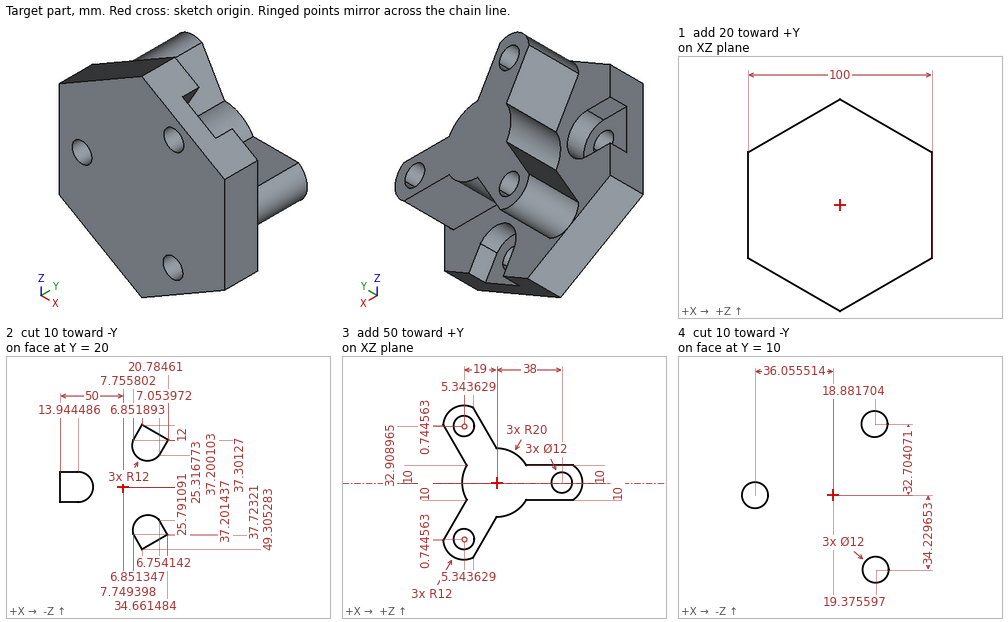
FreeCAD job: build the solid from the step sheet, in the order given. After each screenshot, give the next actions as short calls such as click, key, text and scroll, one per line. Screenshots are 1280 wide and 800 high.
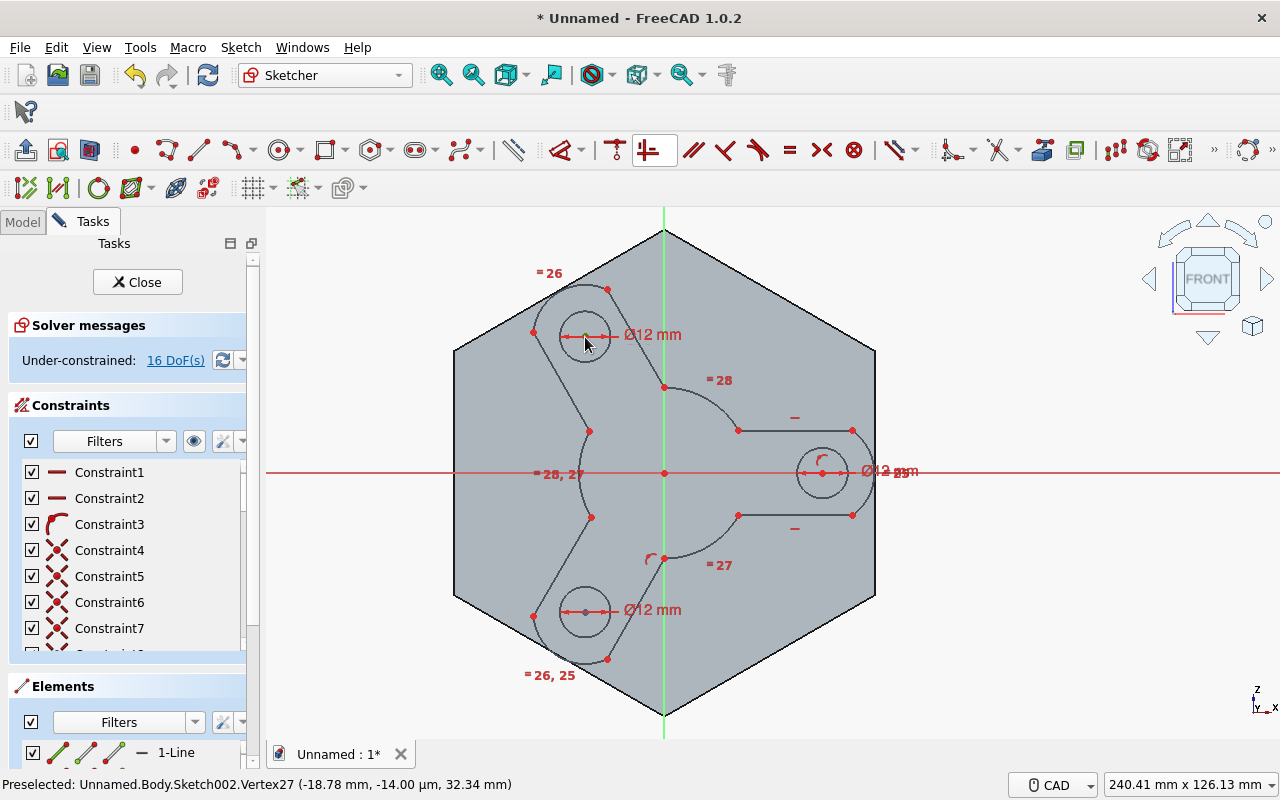
click(353, 473)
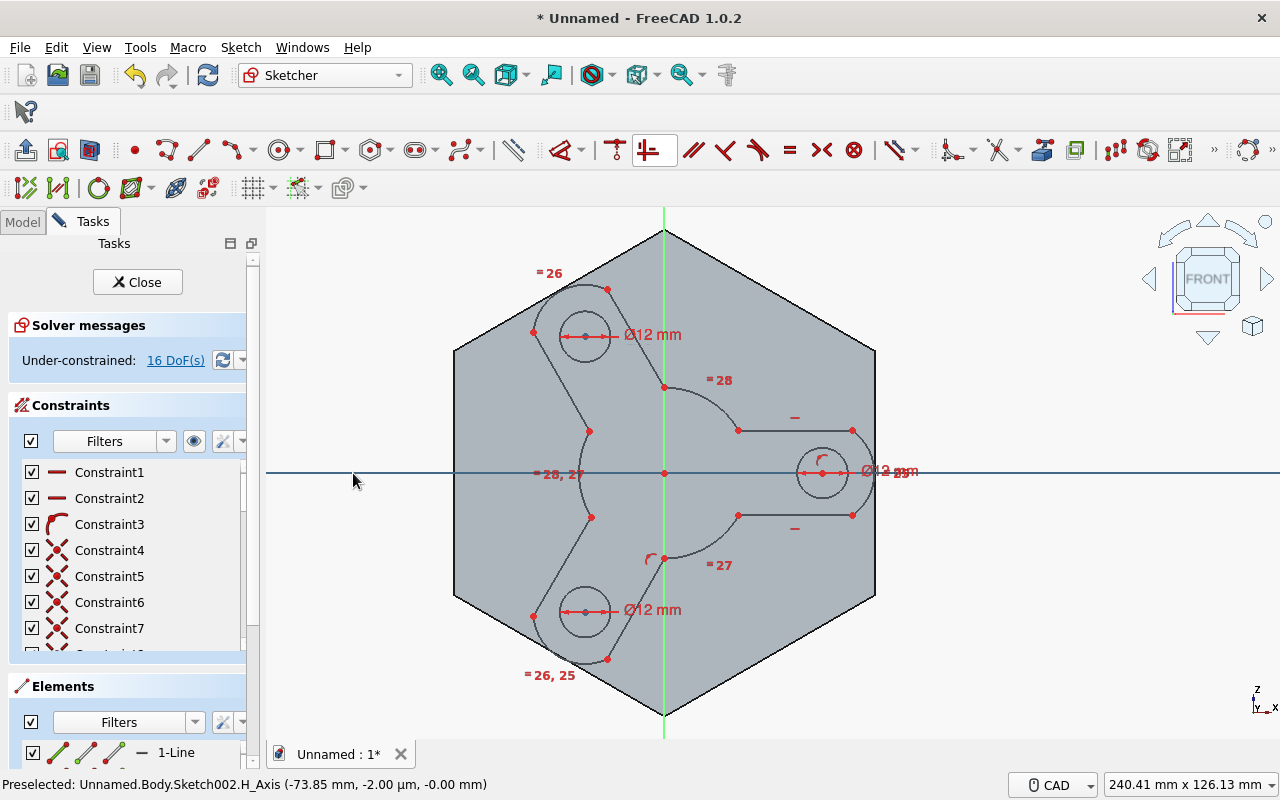
click(822, 150)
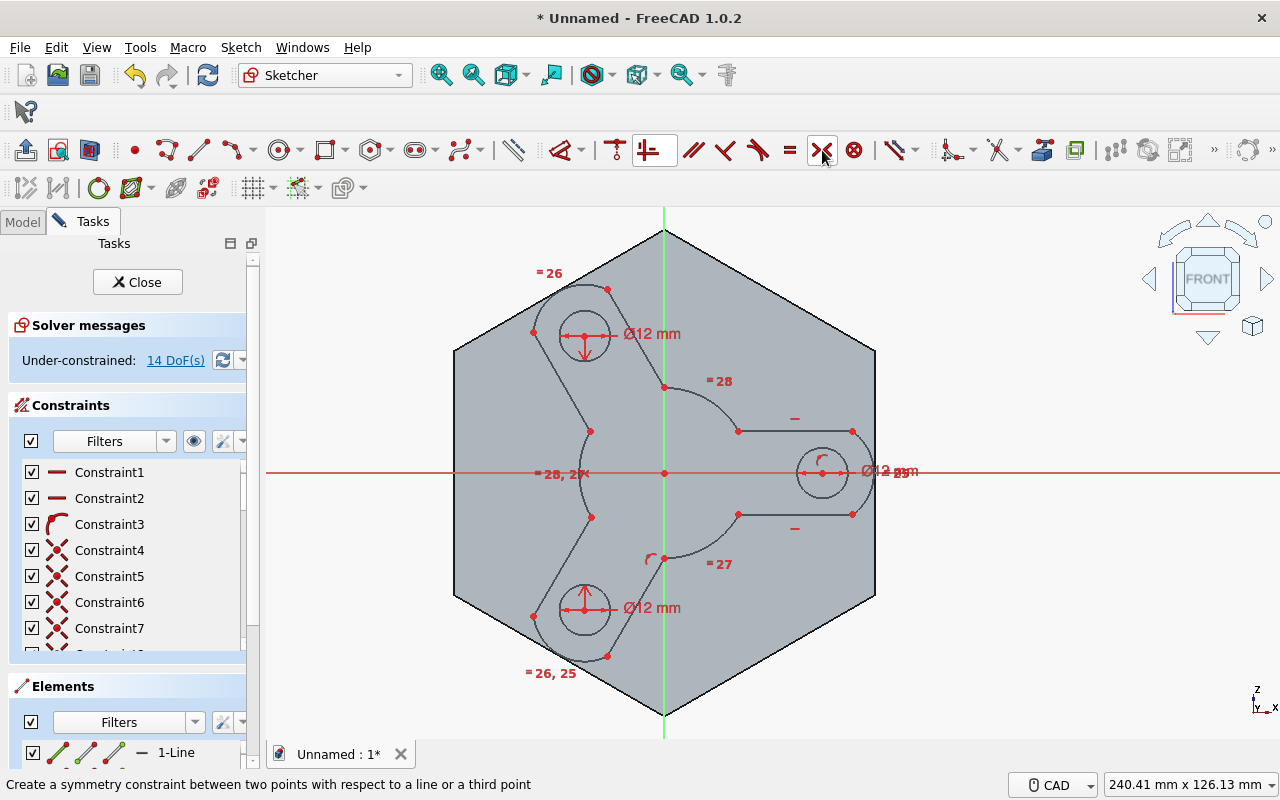
click(560, 150)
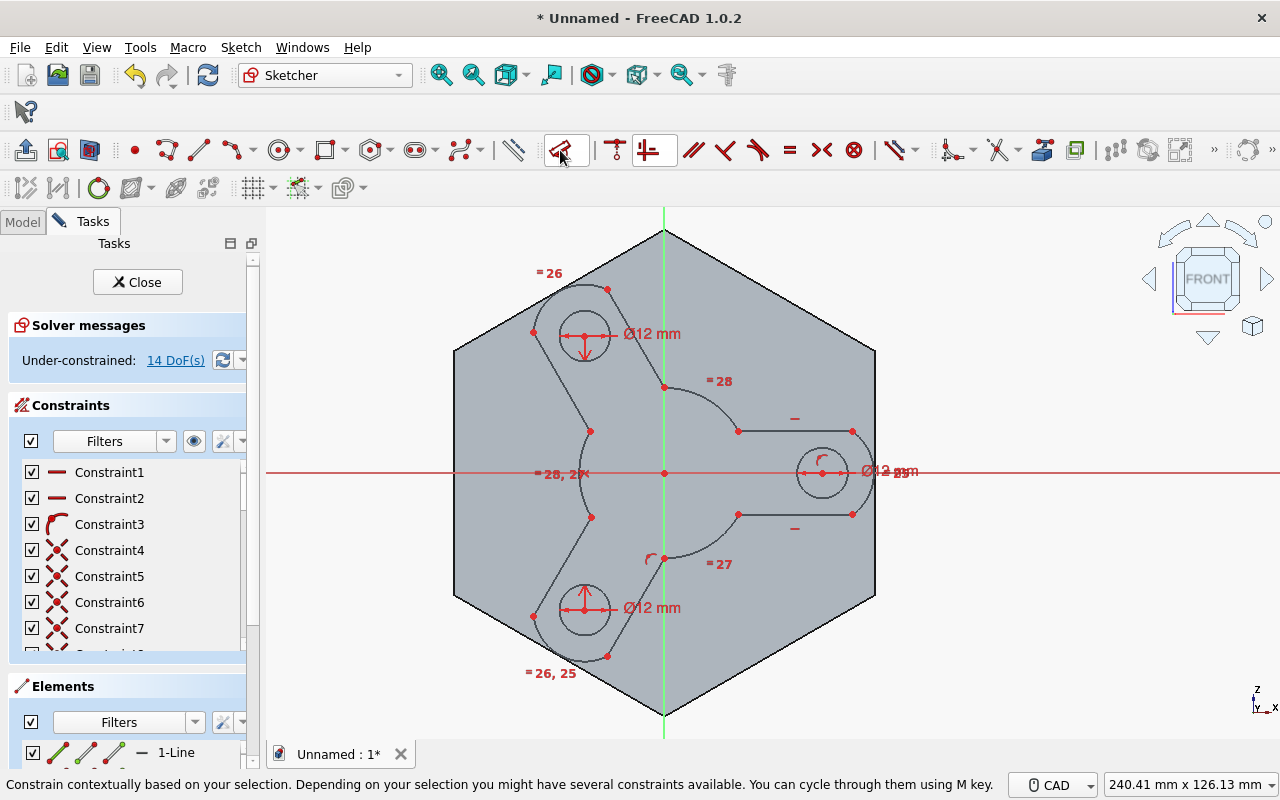
click(870, 492)
click(900, 504)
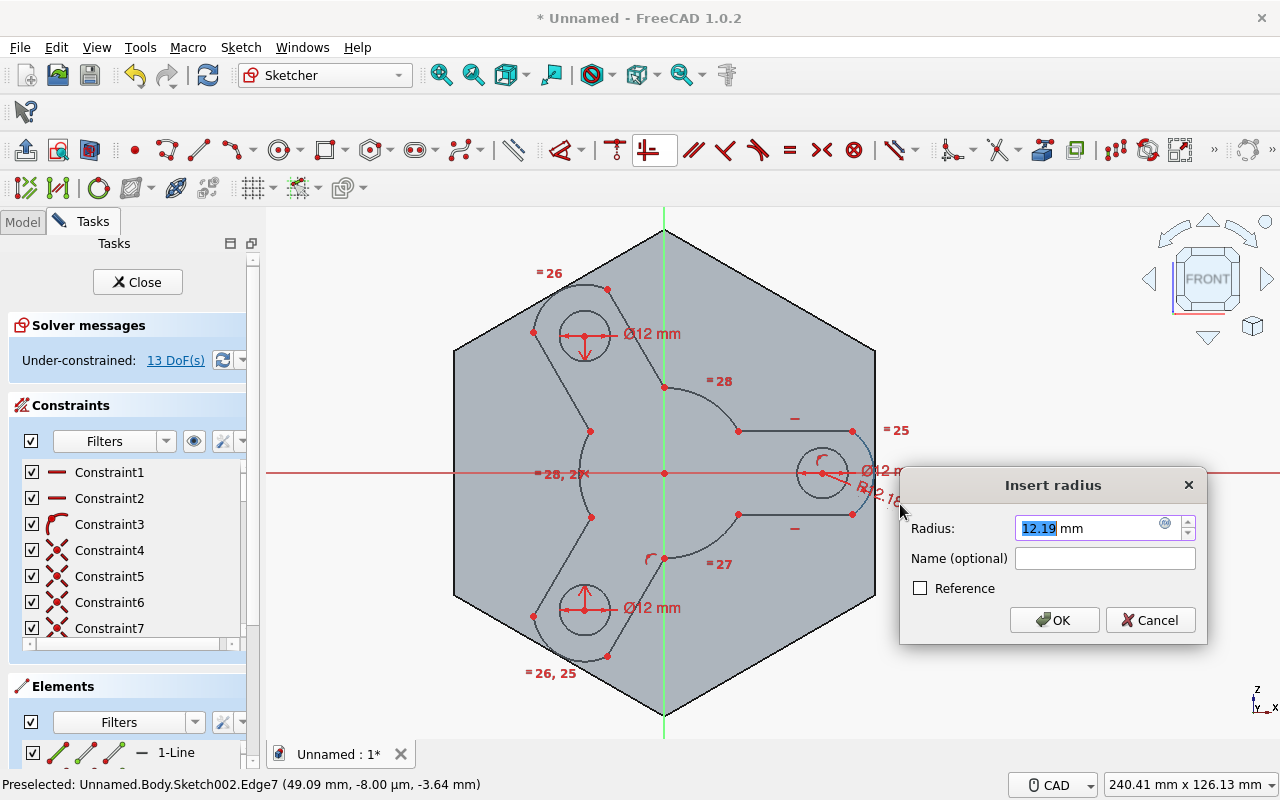
text(12)
key(Return)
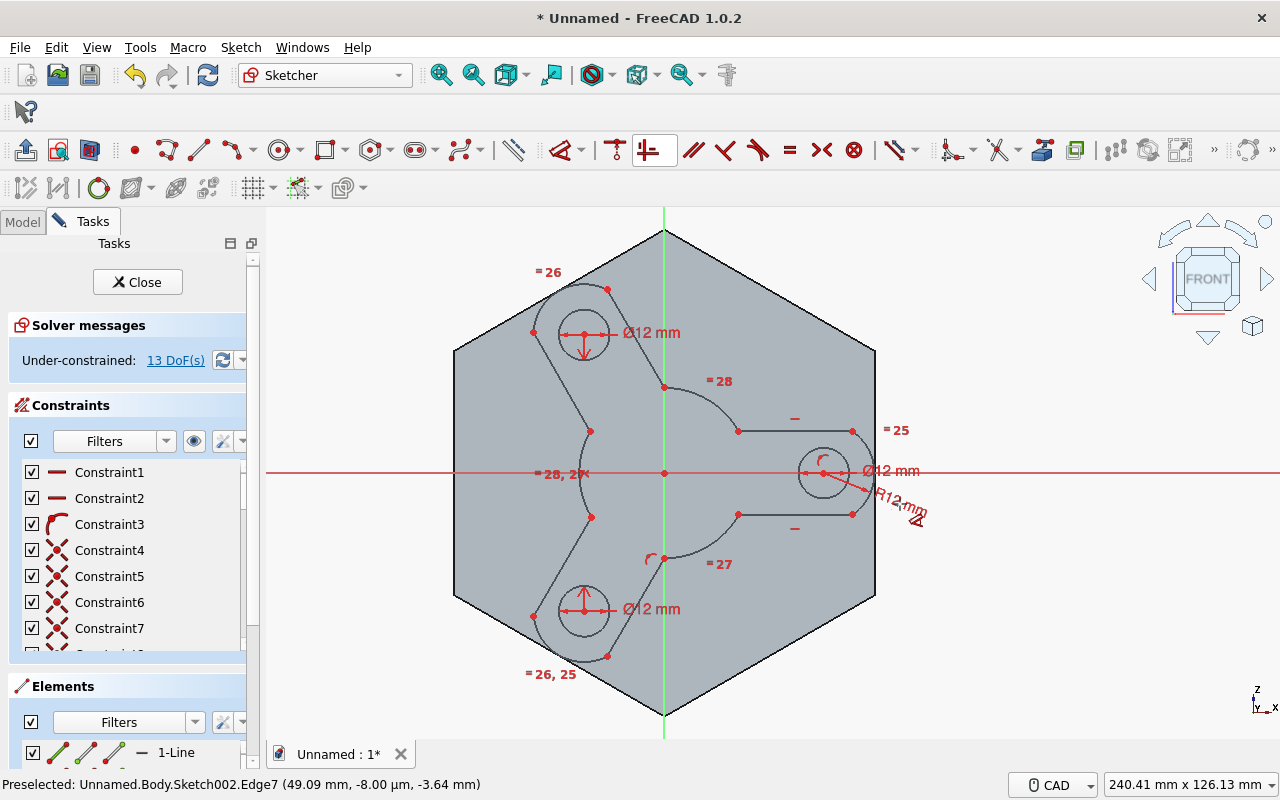
click(691, 554)
click(701, 584)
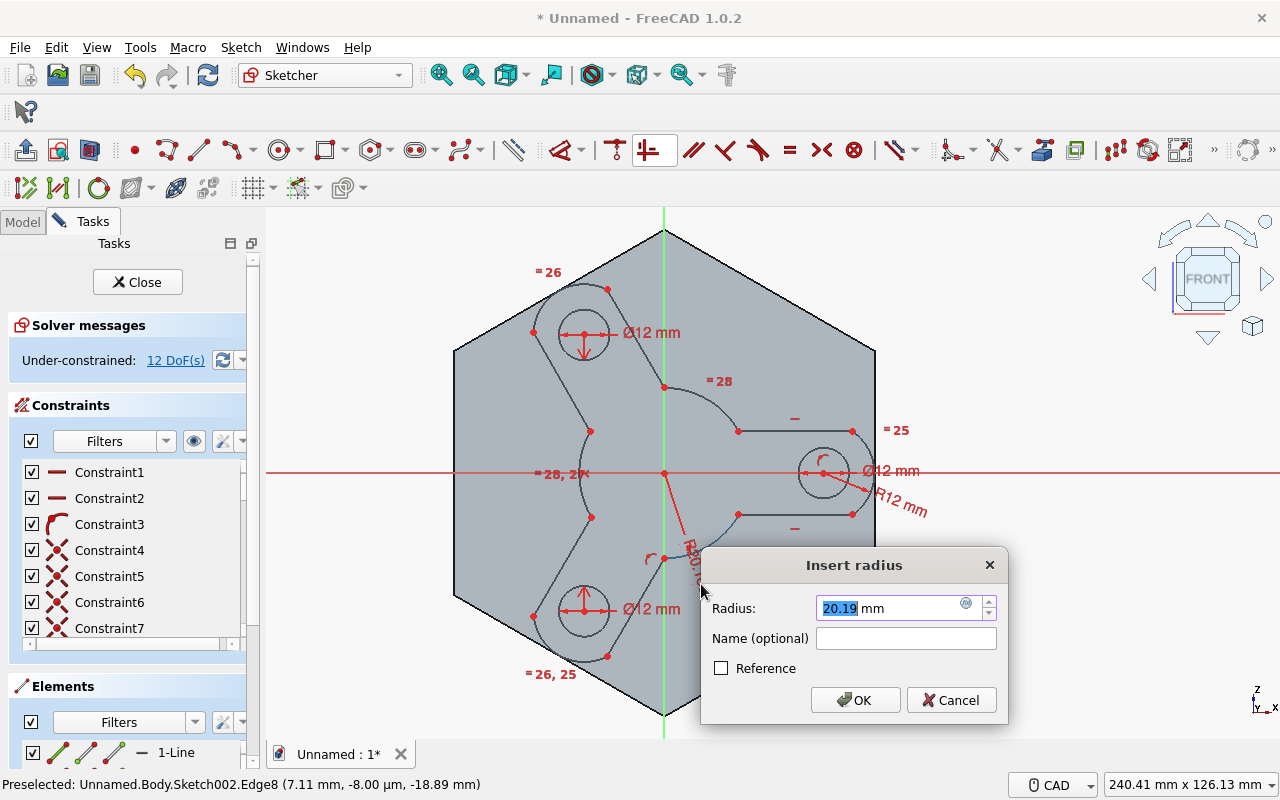
text(20)
key(Return)
key(Escape)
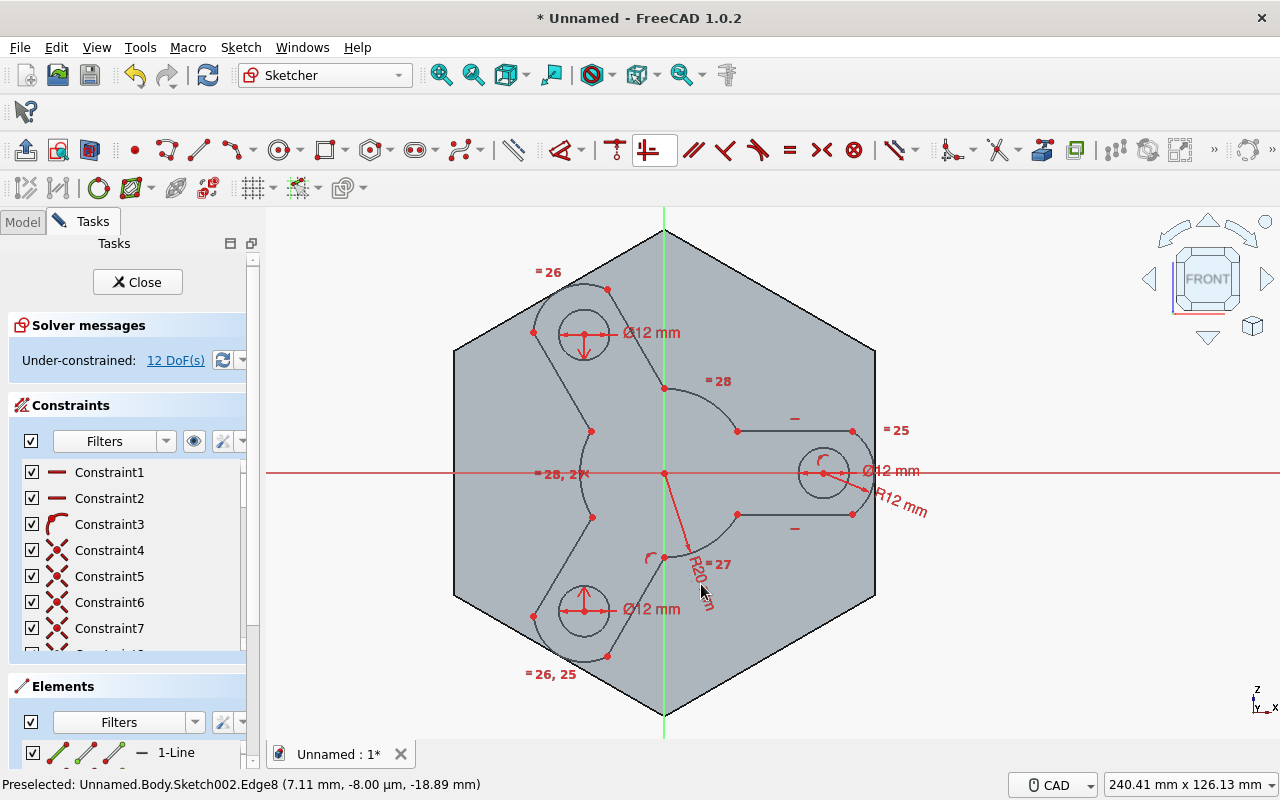
click(664, 389)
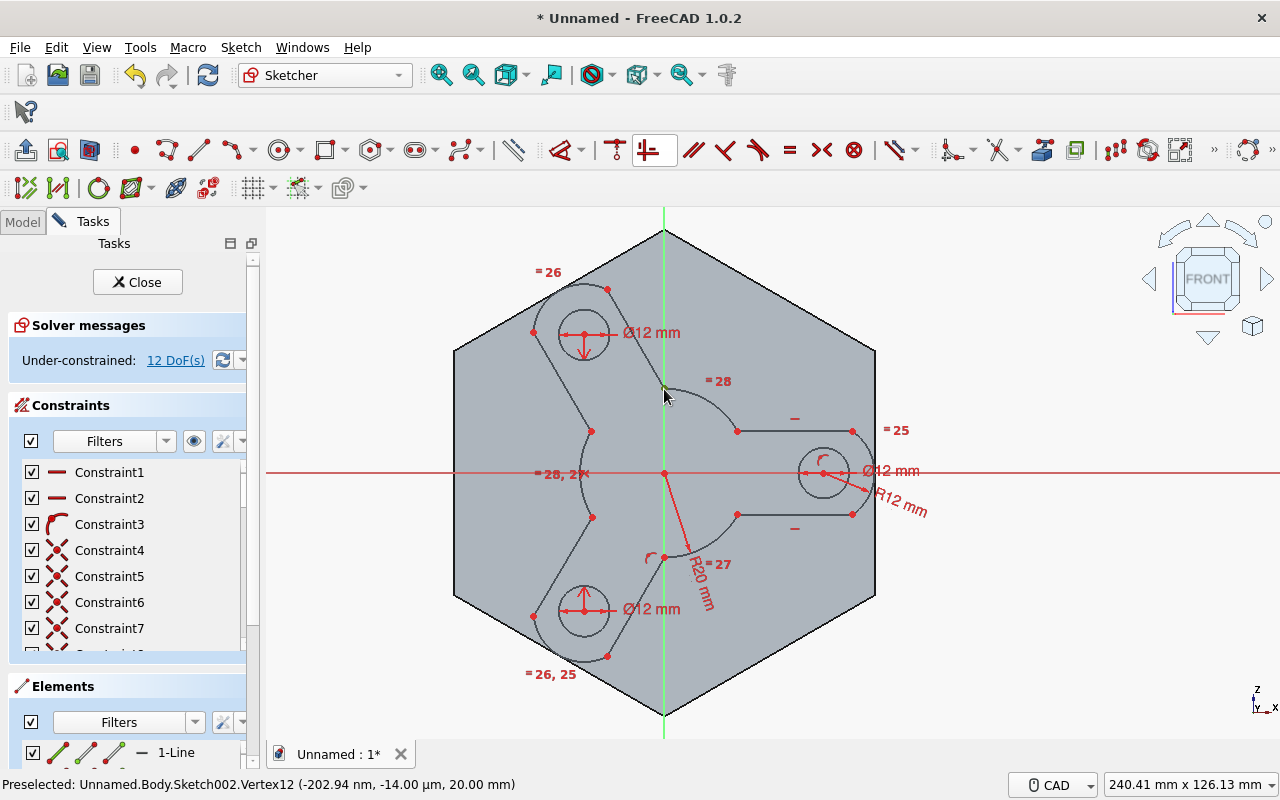
click(664, 677)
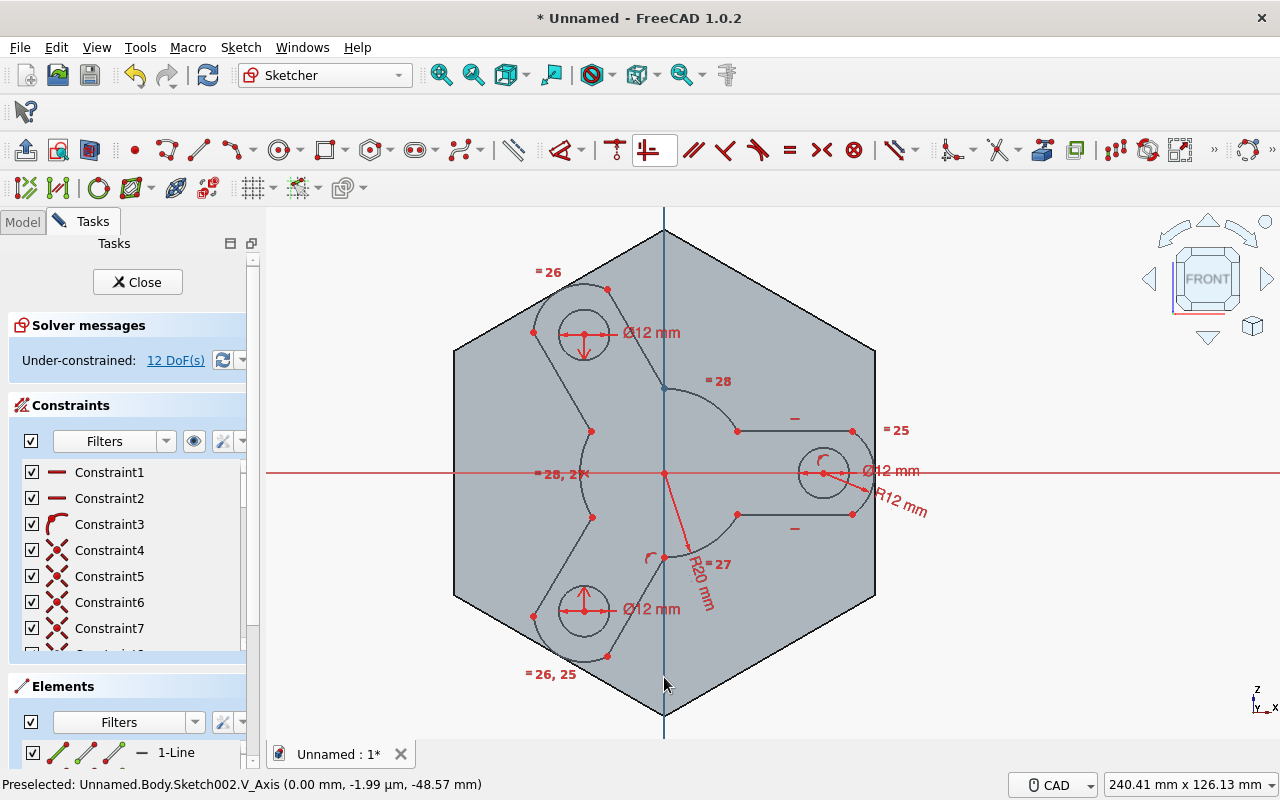
click(616, 150)